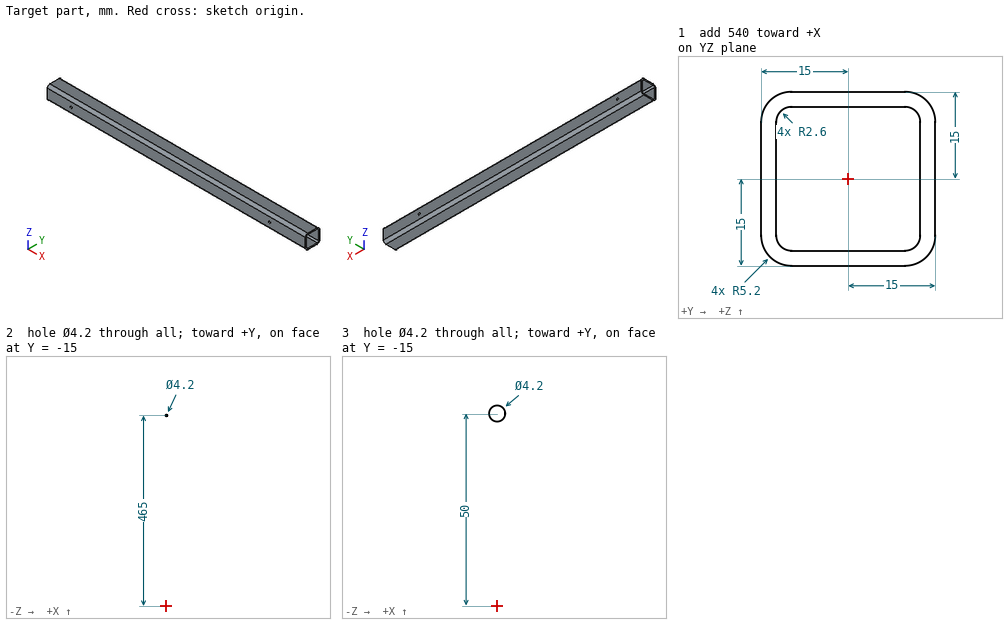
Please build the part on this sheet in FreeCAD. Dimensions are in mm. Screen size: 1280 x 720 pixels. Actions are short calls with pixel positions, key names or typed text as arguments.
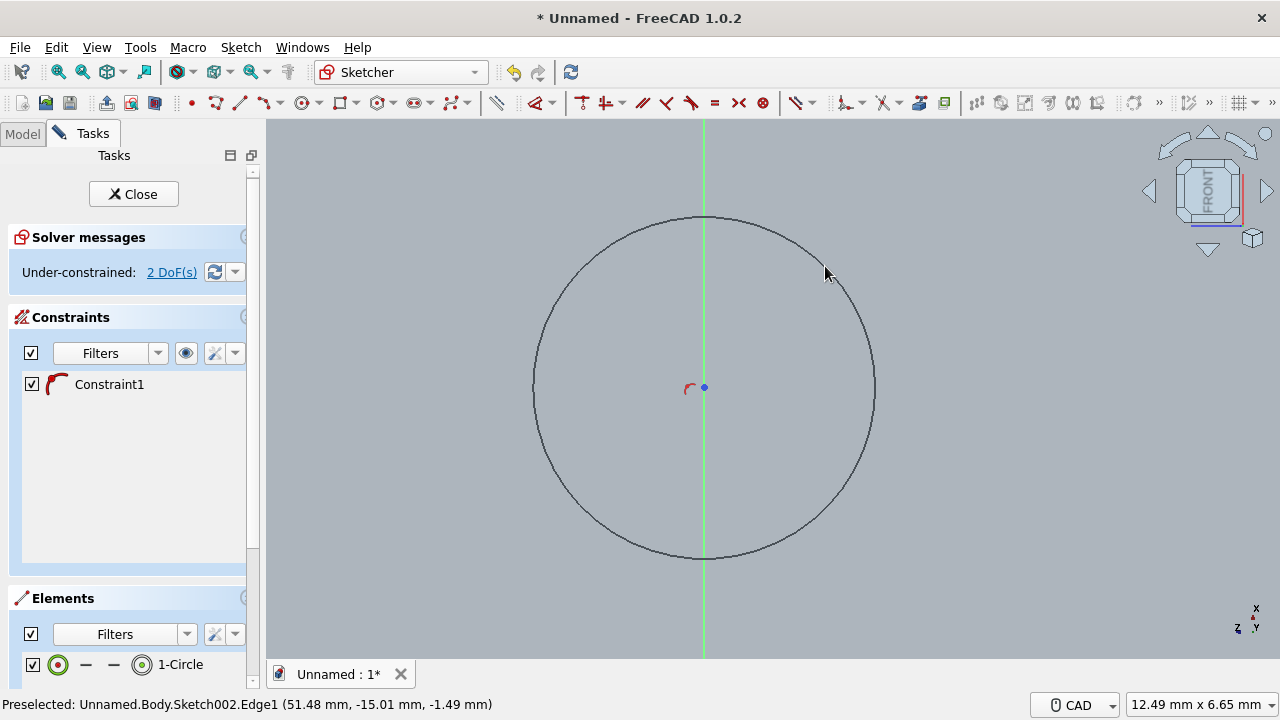
click(536, 104)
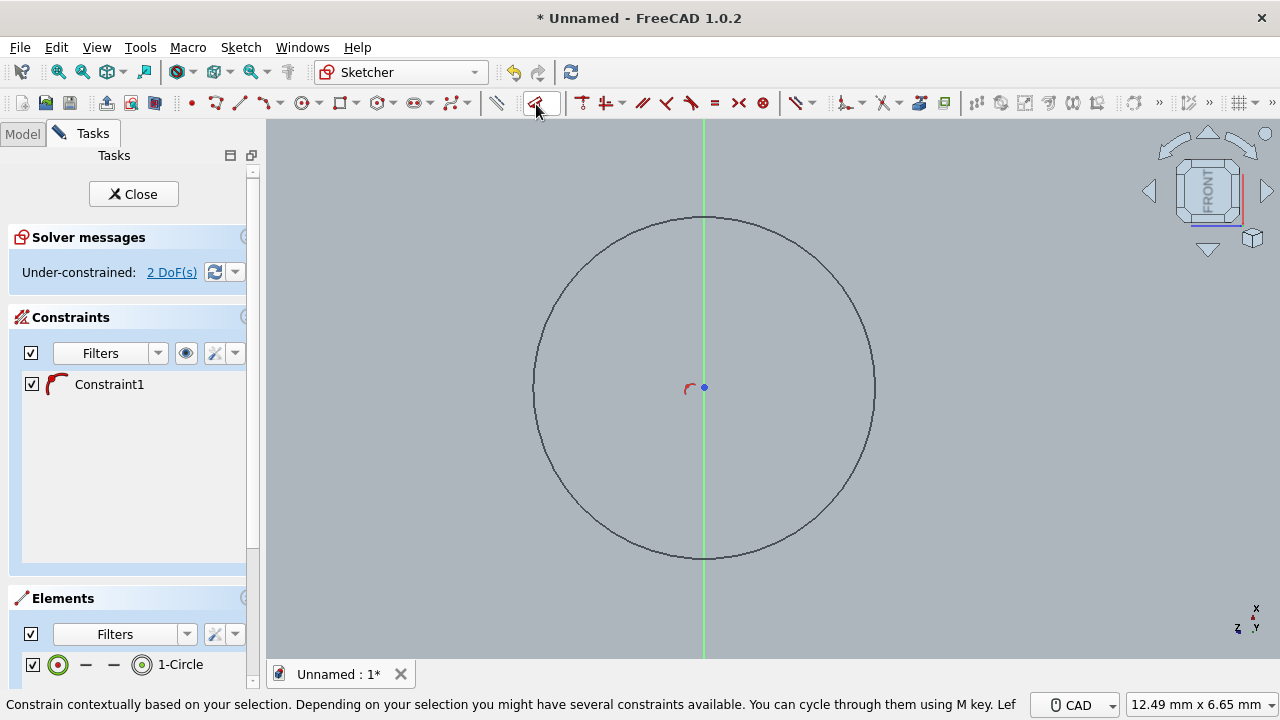
click(825, 267)
click(848, 244)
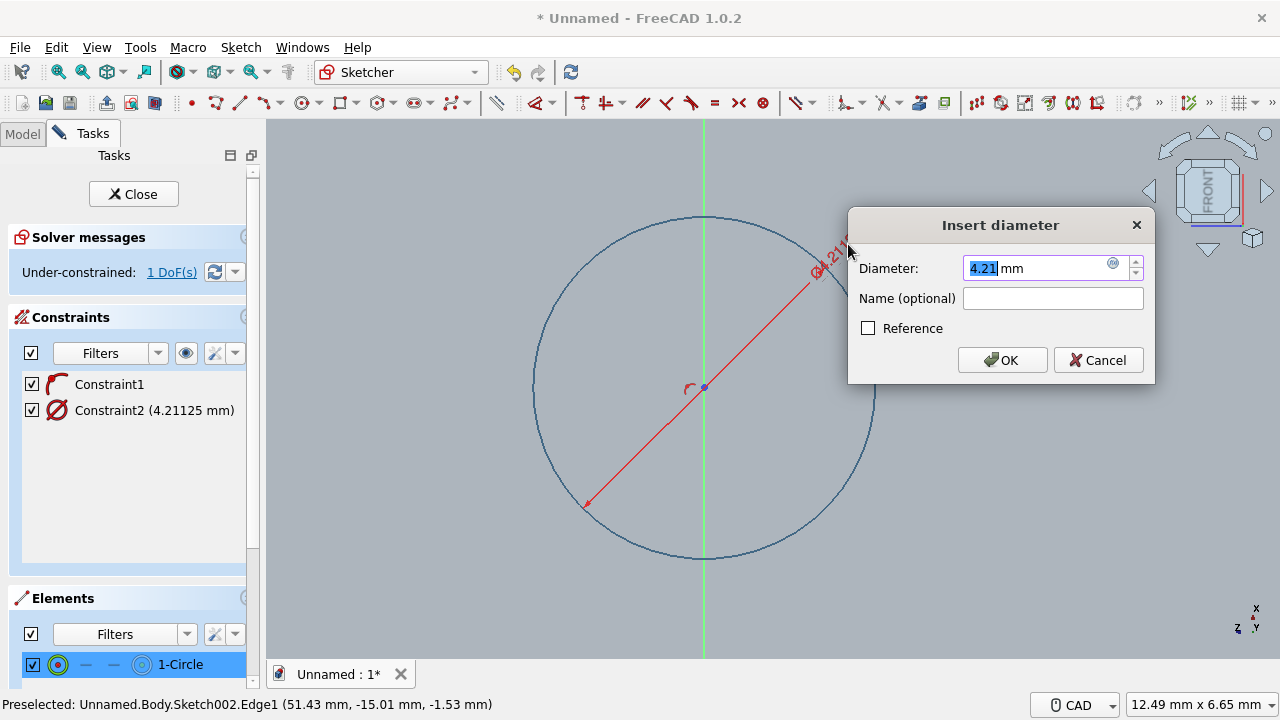
text(4.2)
key(Return)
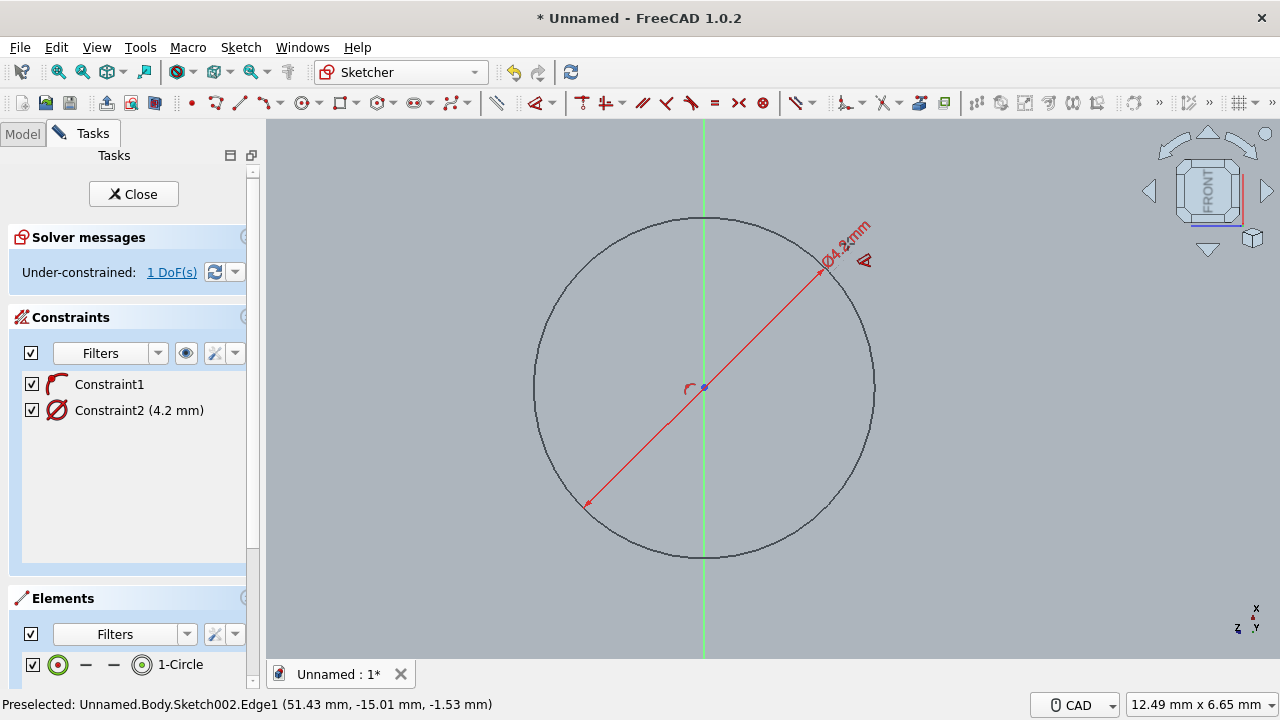
click(704, 388)
click(738, 510)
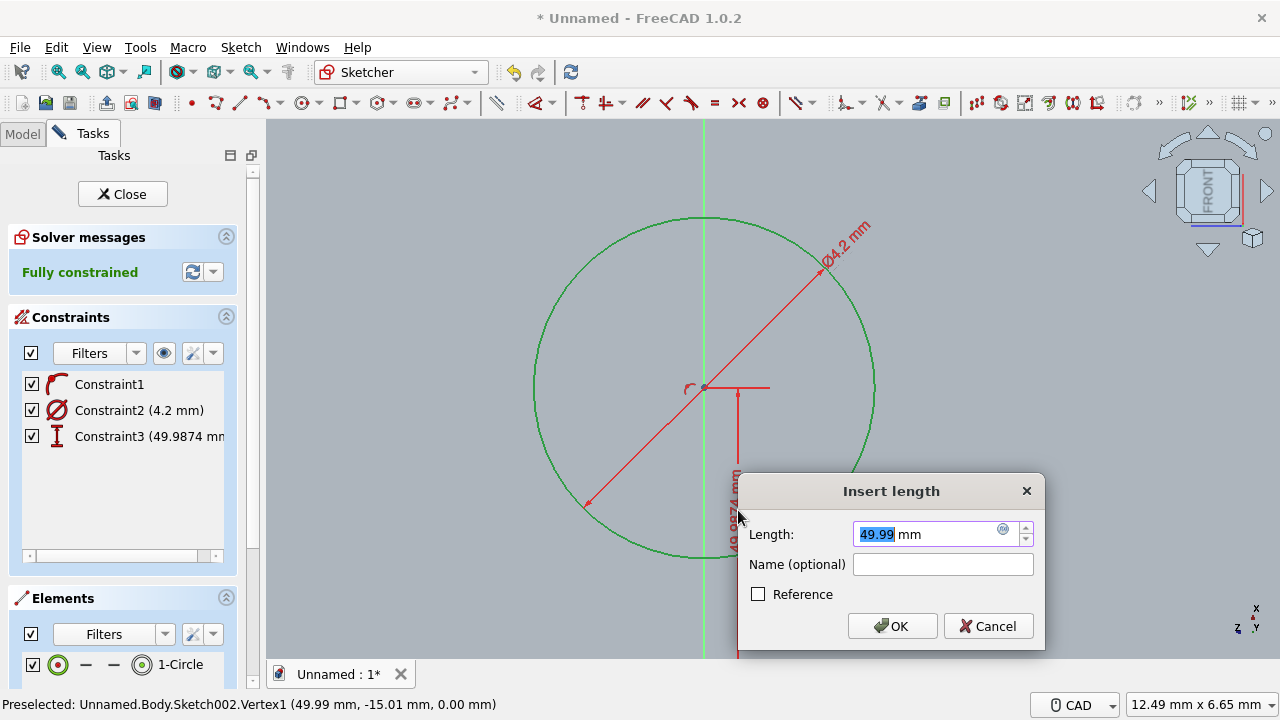
text(50)
key(Return)
key(Escape)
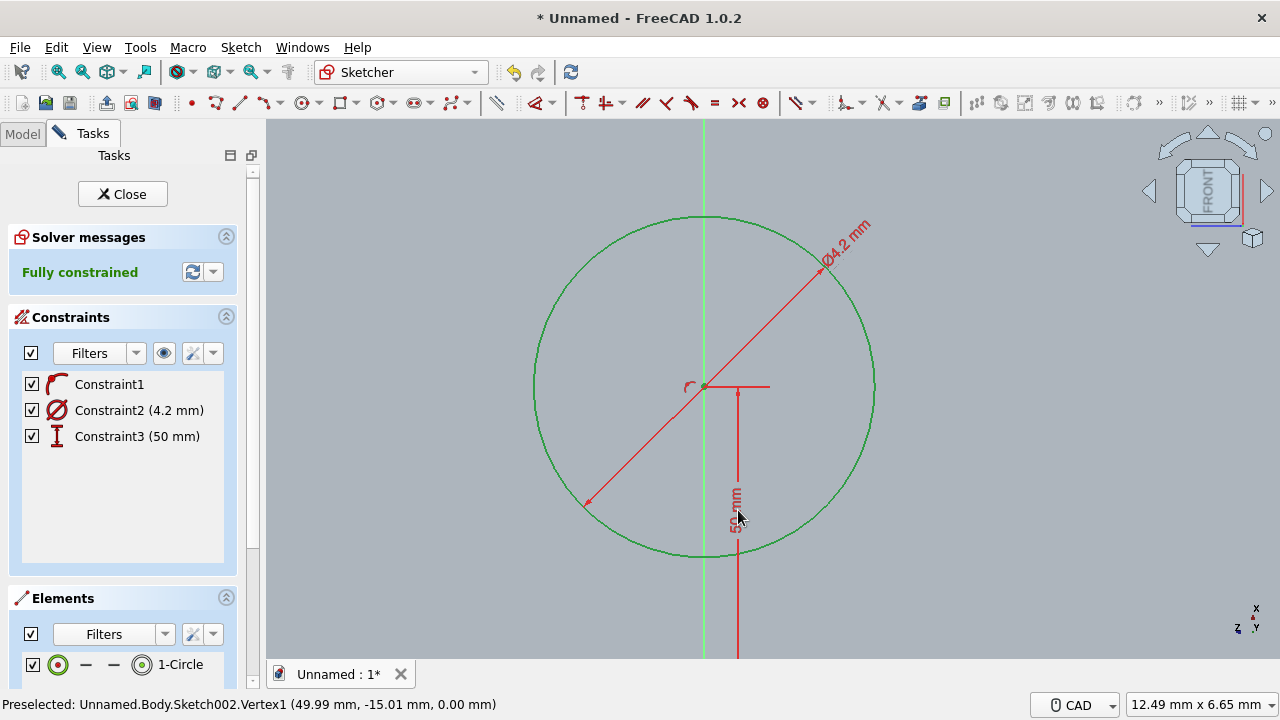
click(123, 194)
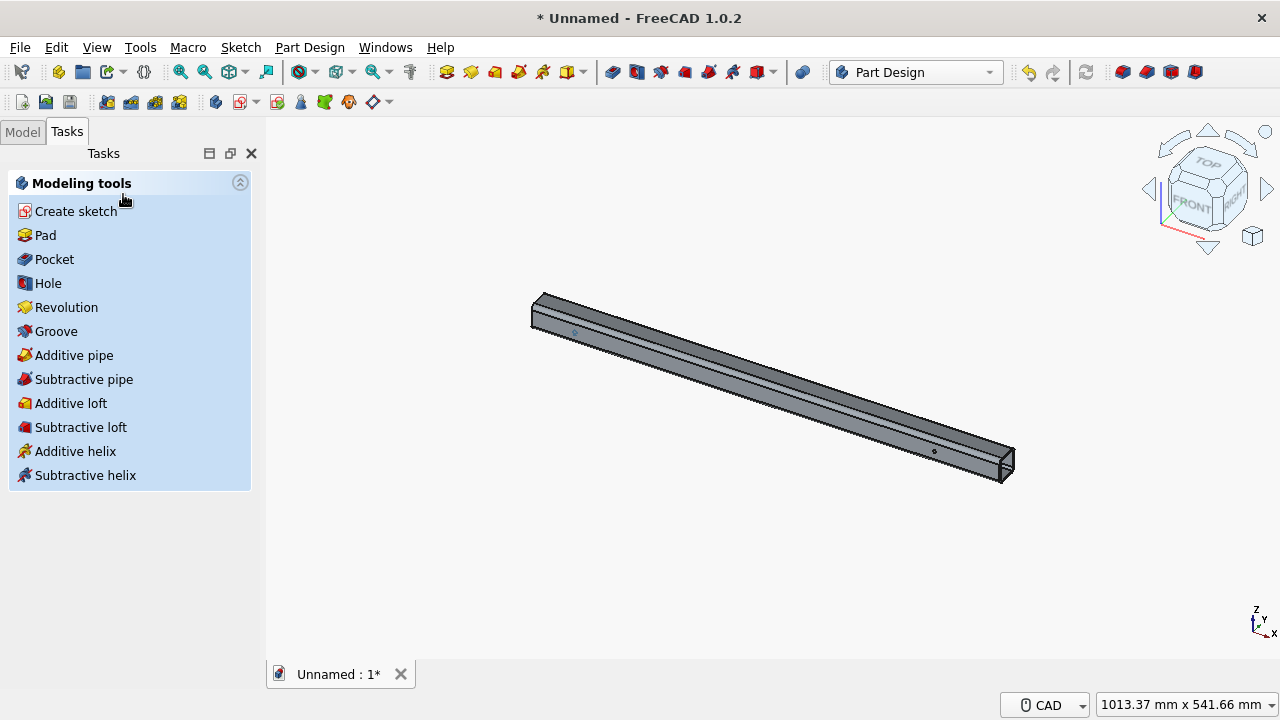
click(638, 72)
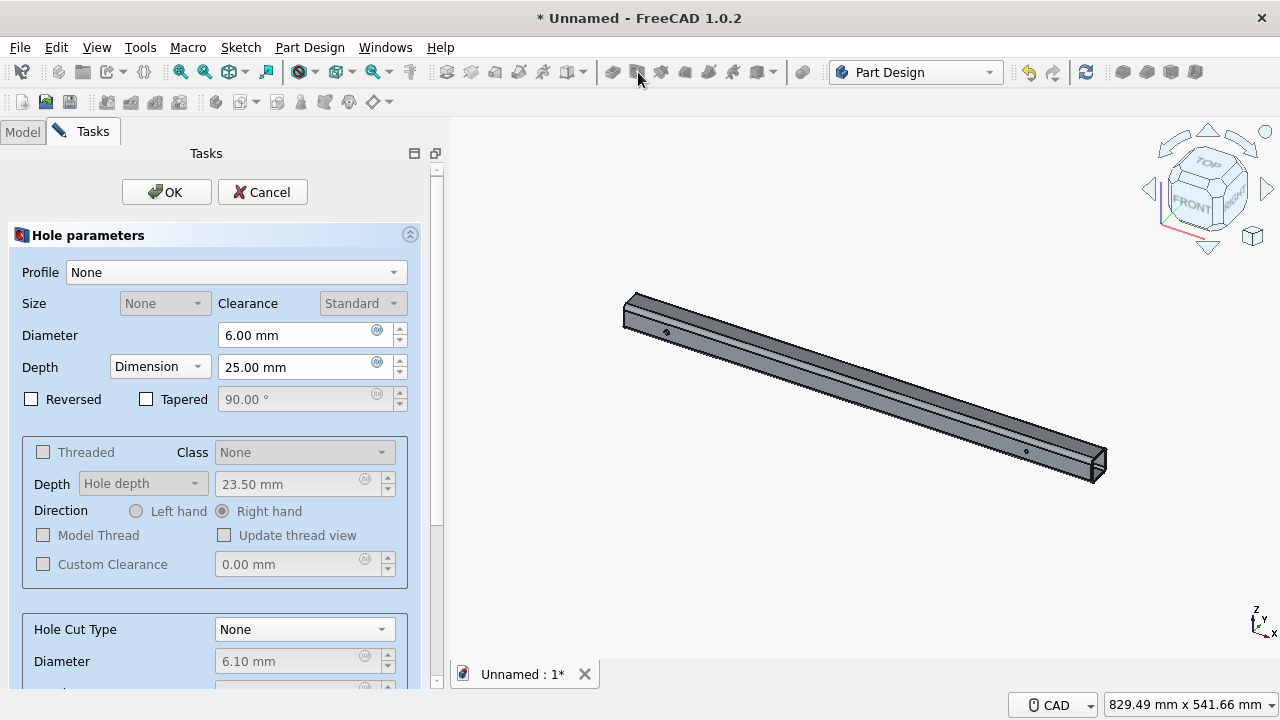
triple_click(305, 335)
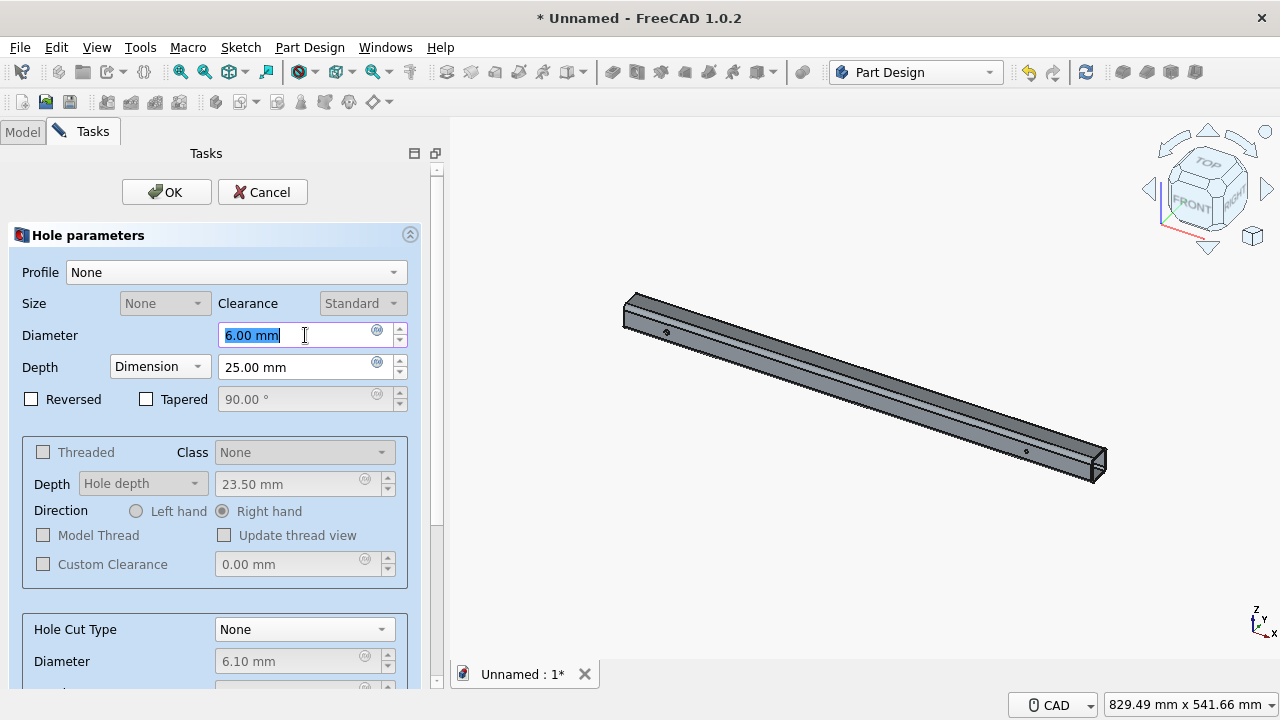
text(4.2)
key(Tab)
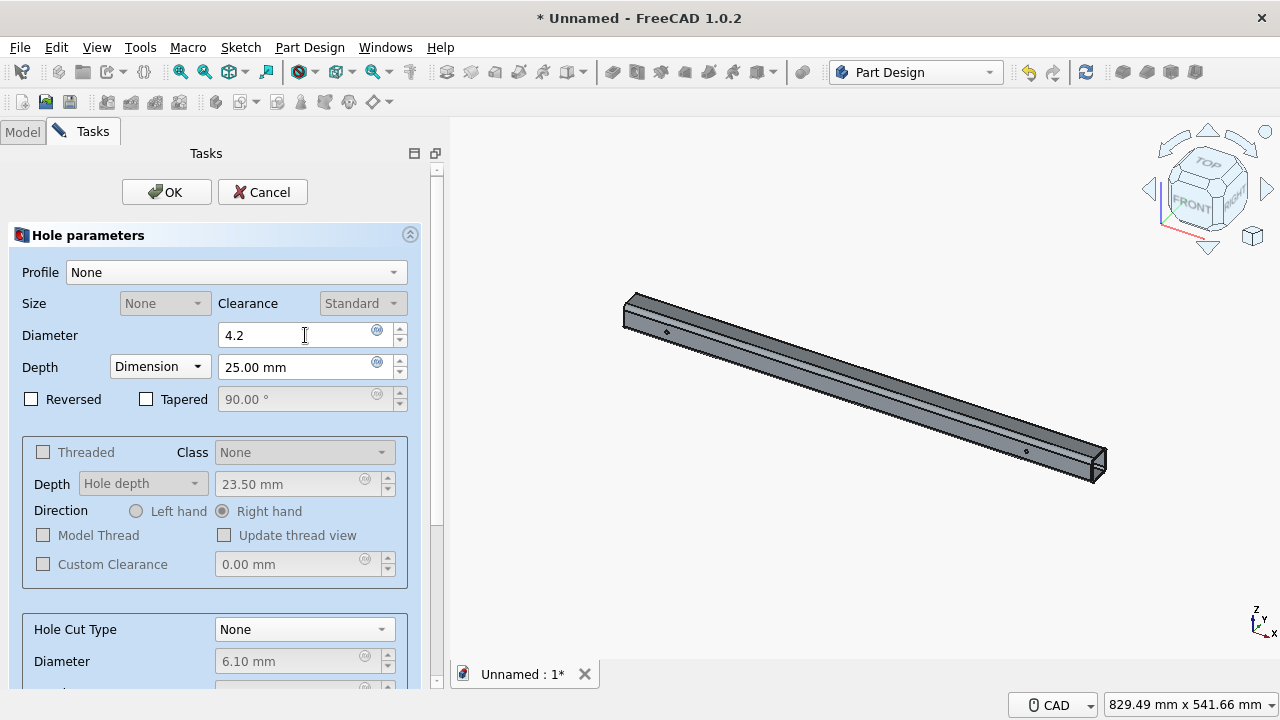
click(161, 366)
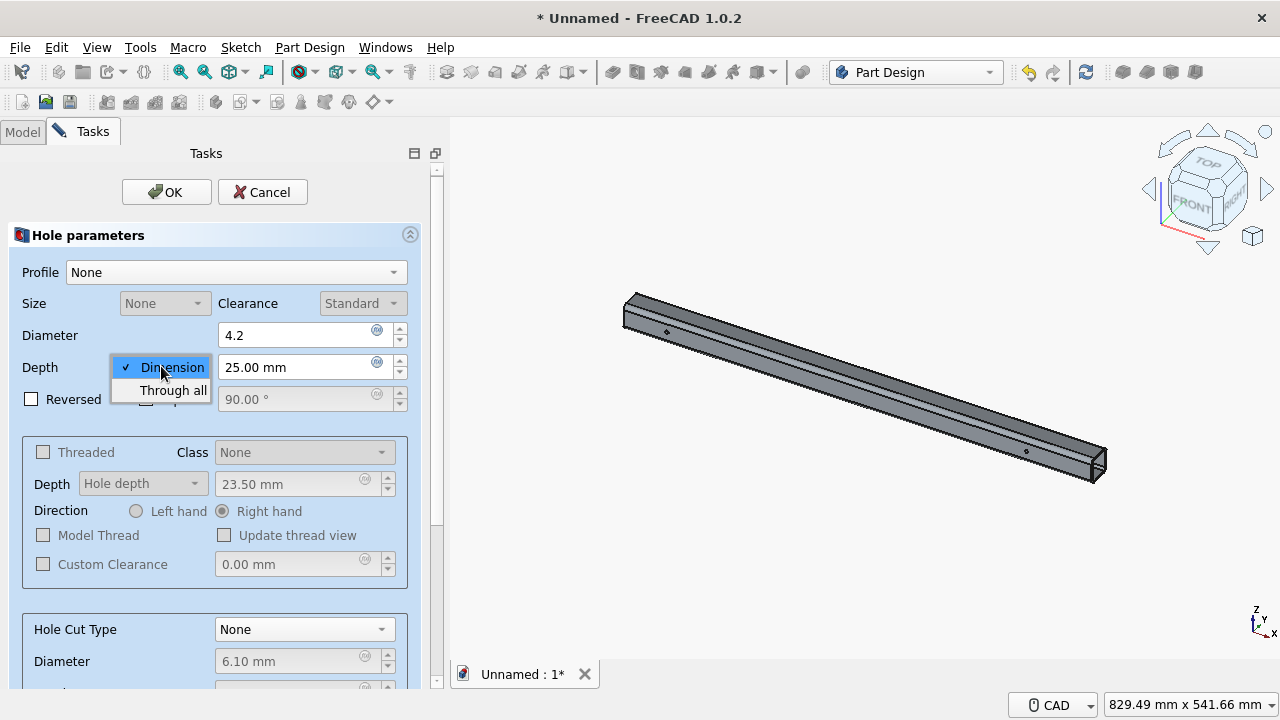
click(160, 390)